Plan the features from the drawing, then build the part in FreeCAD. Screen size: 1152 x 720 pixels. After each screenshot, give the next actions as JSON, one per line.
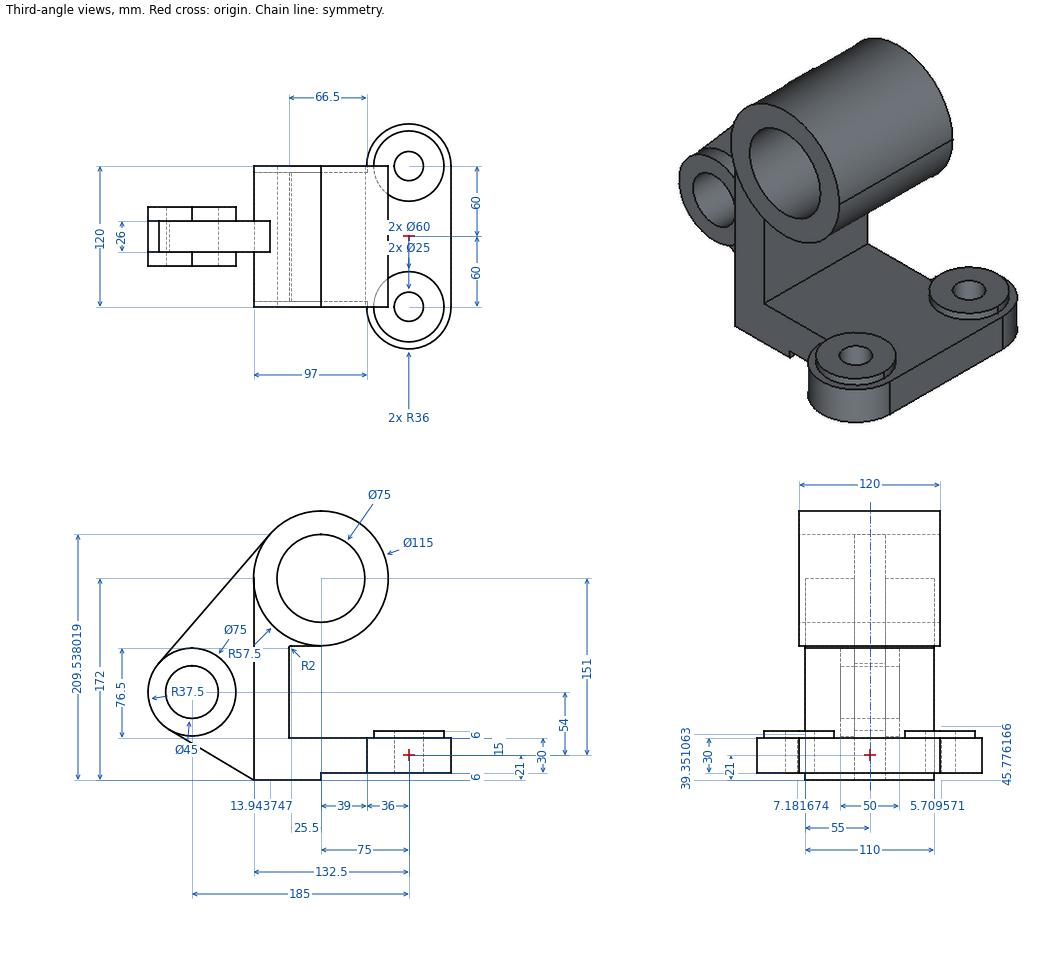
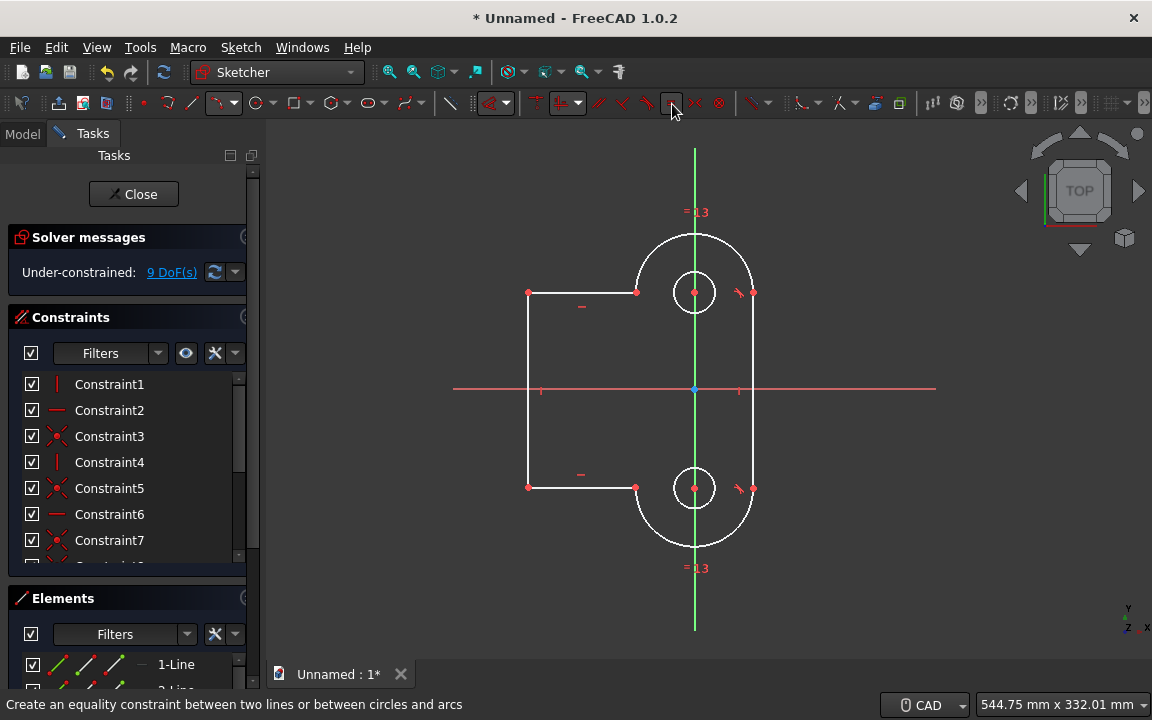
{"action": "left_click", "coordinate": [709, 474]}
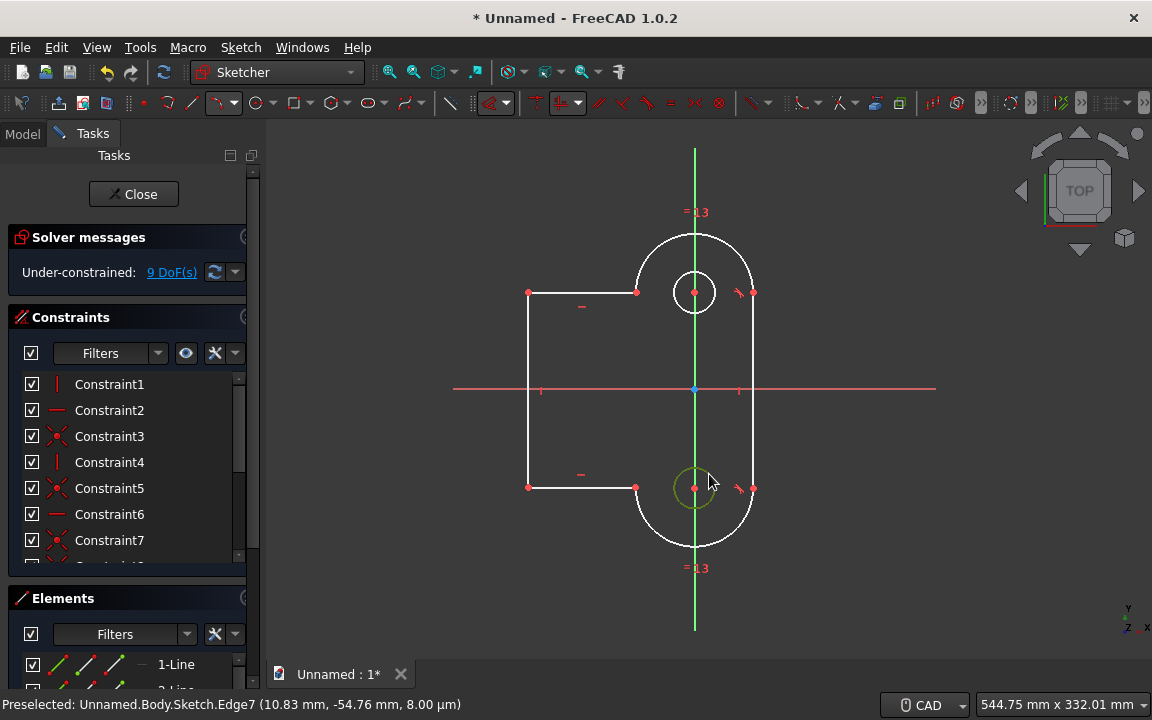
{"action": "left_click", "coordinate": [709, 278]}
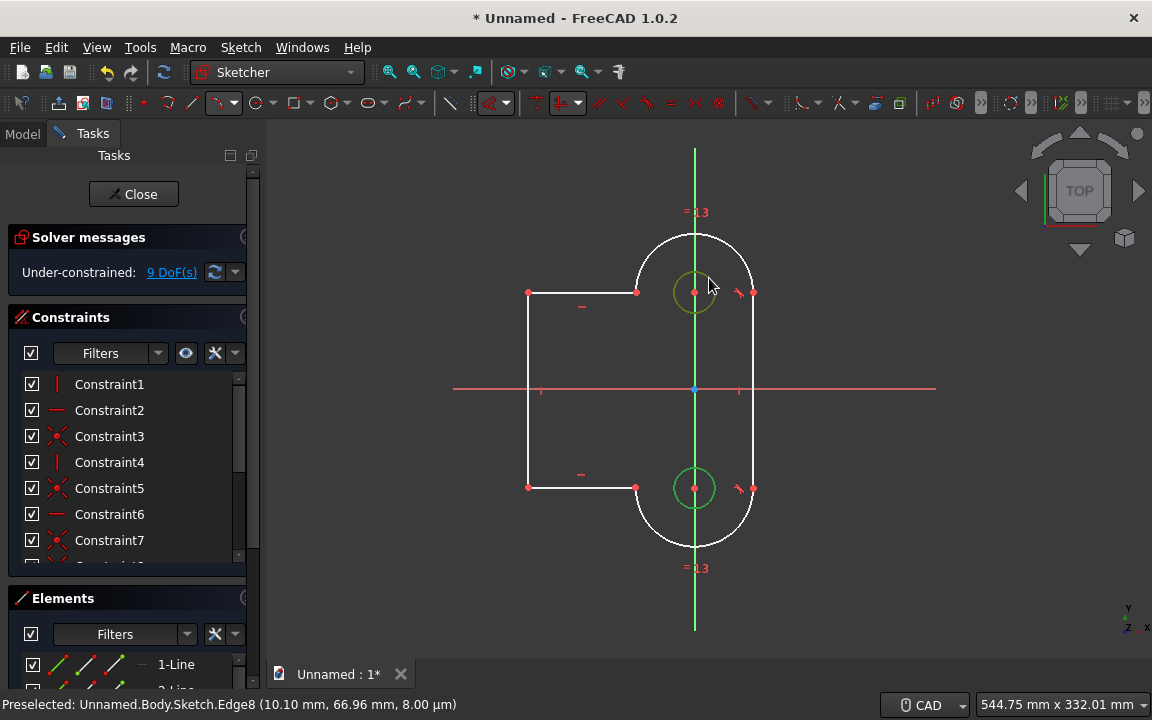
{"action": "left_click", "coordinate": [672, 104]}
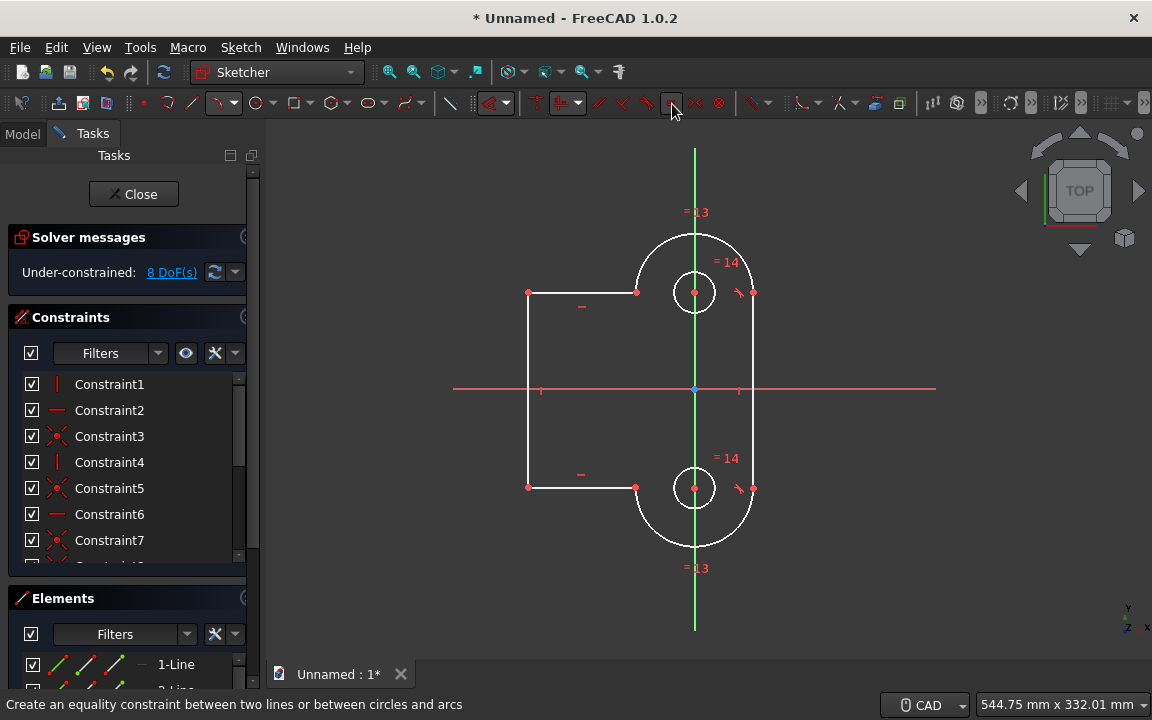
{"action": "left_click", "coordinate": [694, 293]}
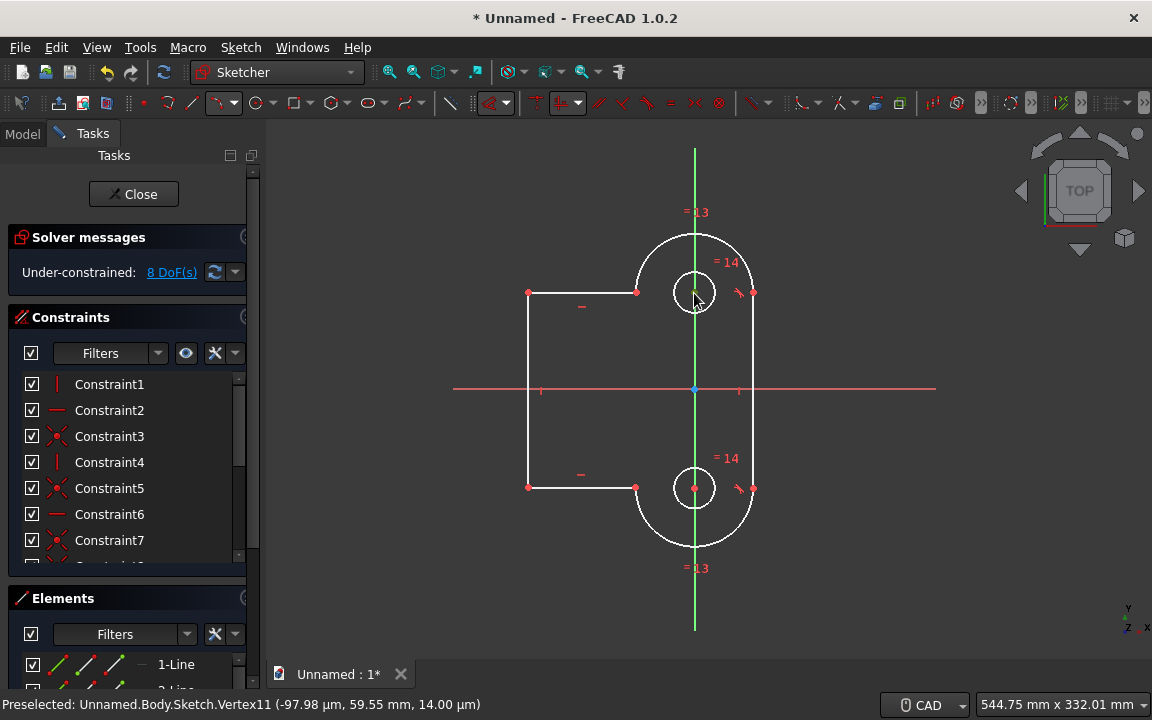
{"action": "left_click", "coordinate": [695, 596]}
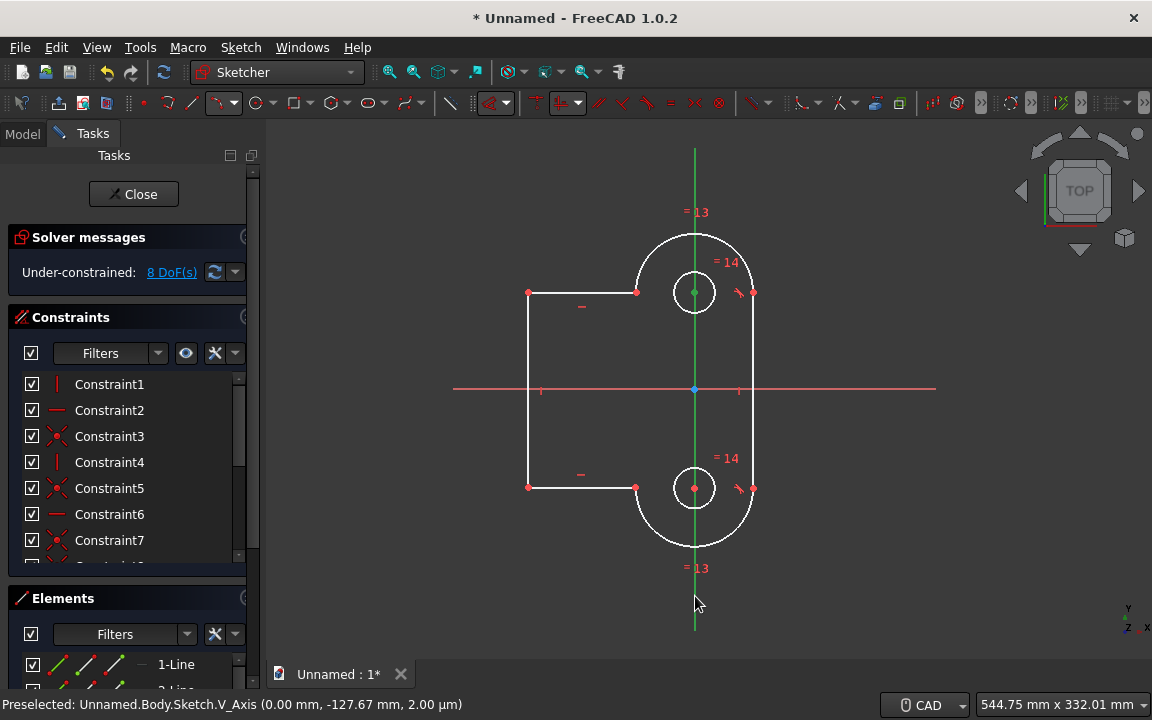
{"action": "key", "text": "c"}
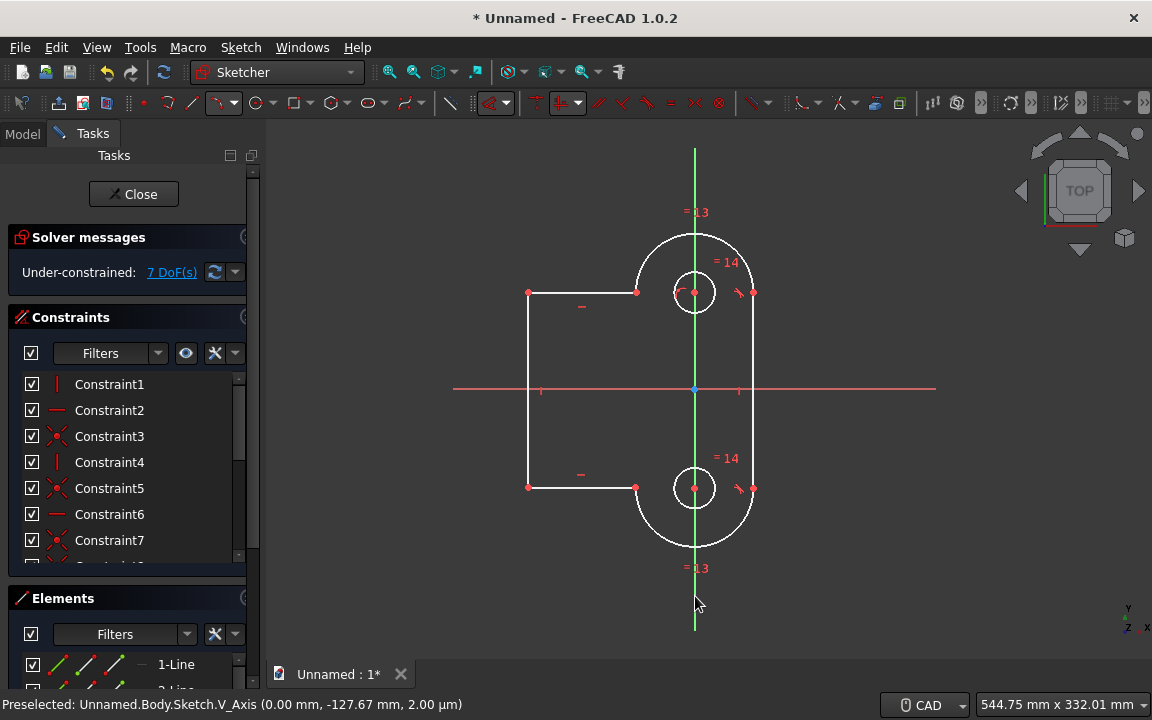
{"action": "left_click", "coordinate": [729, 245]}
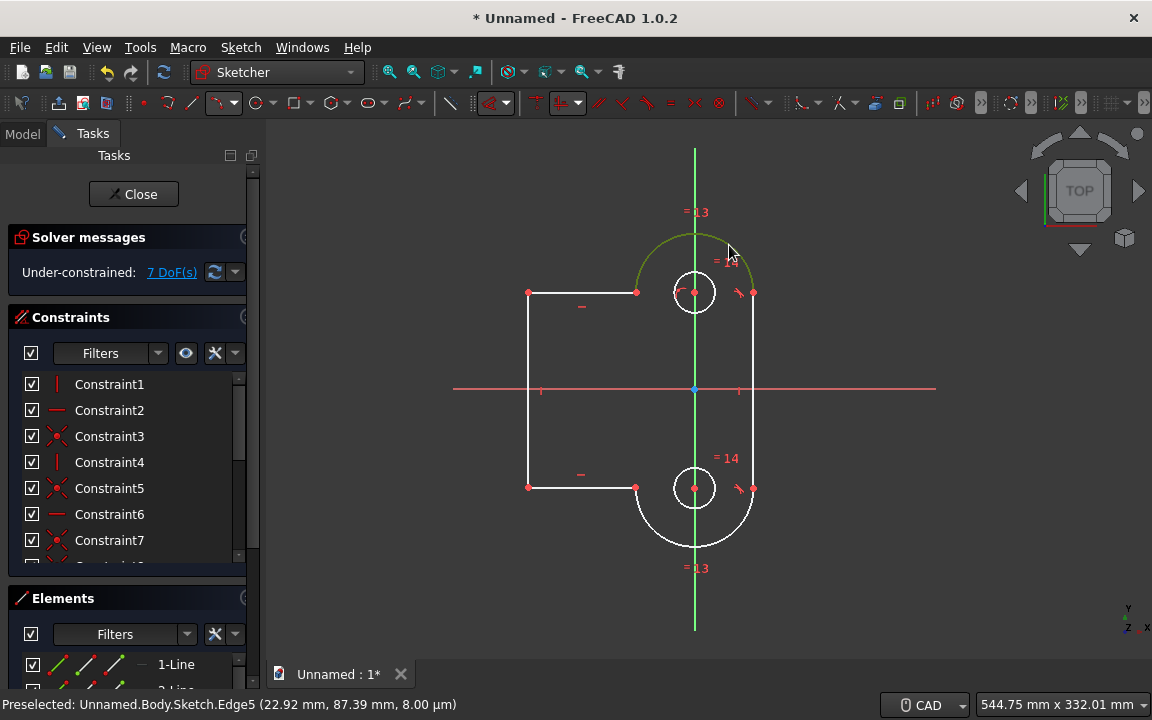
{"action": "key", "text": "k r"}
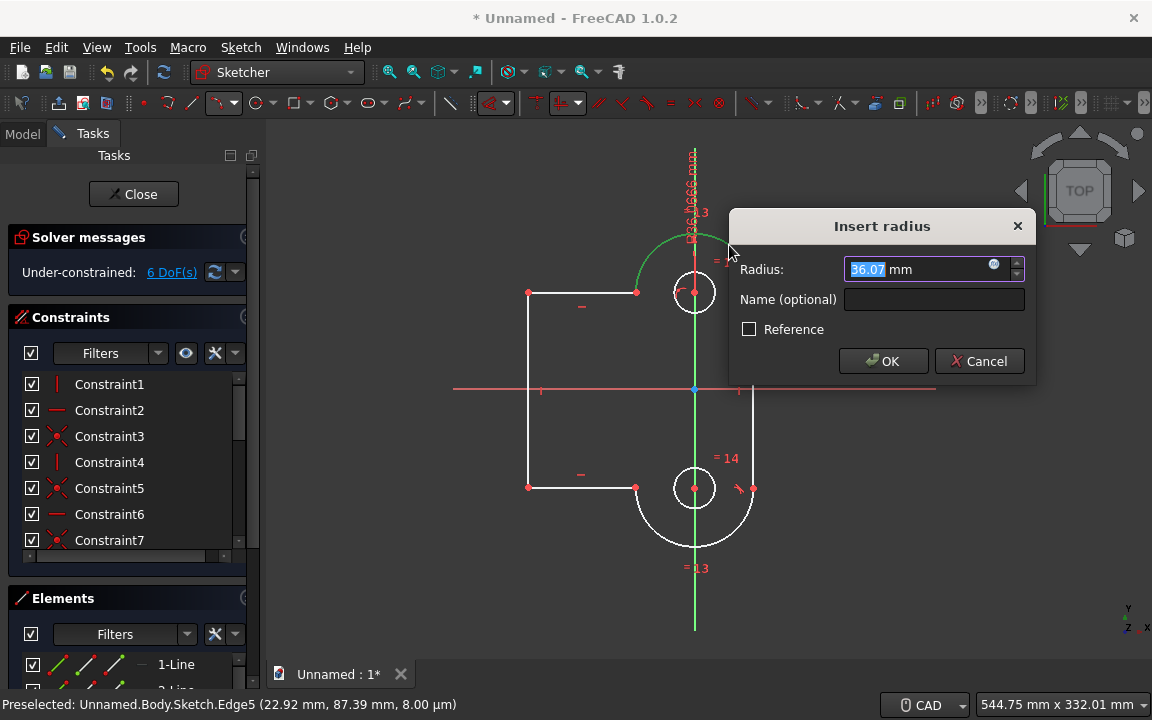
{"action": "type", "text": "36"}
{"action": "key", "text": "Return"}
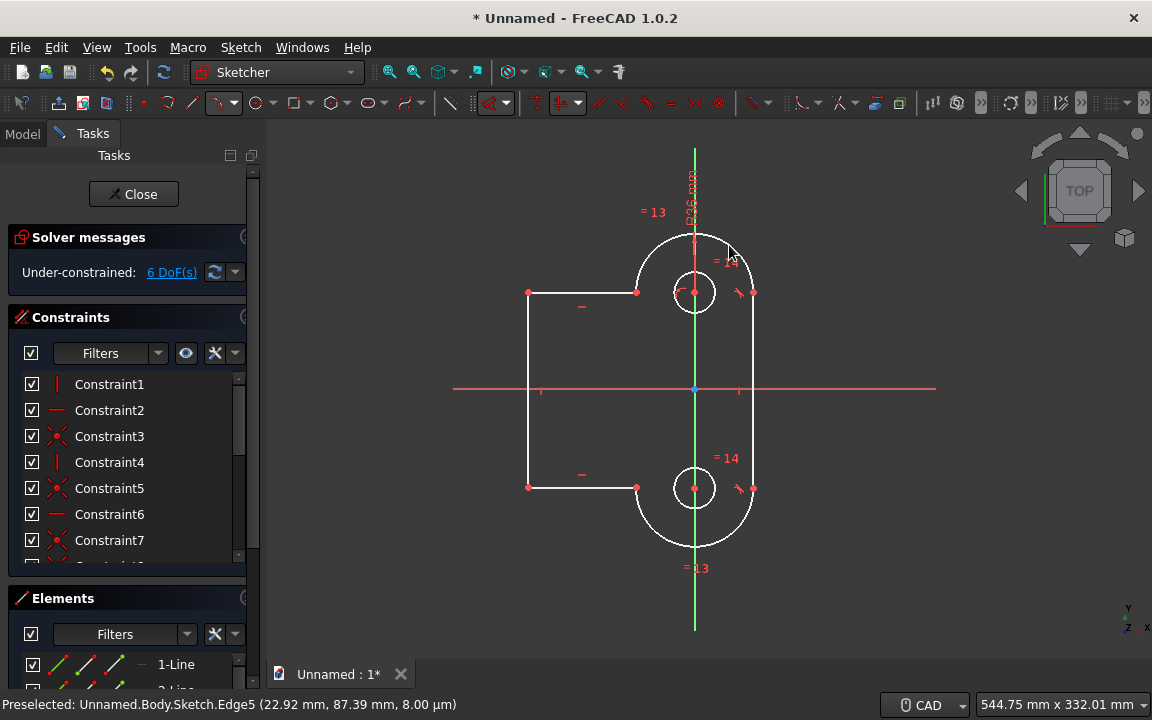
{"action": "left_click", "coordinate": [709, 474]}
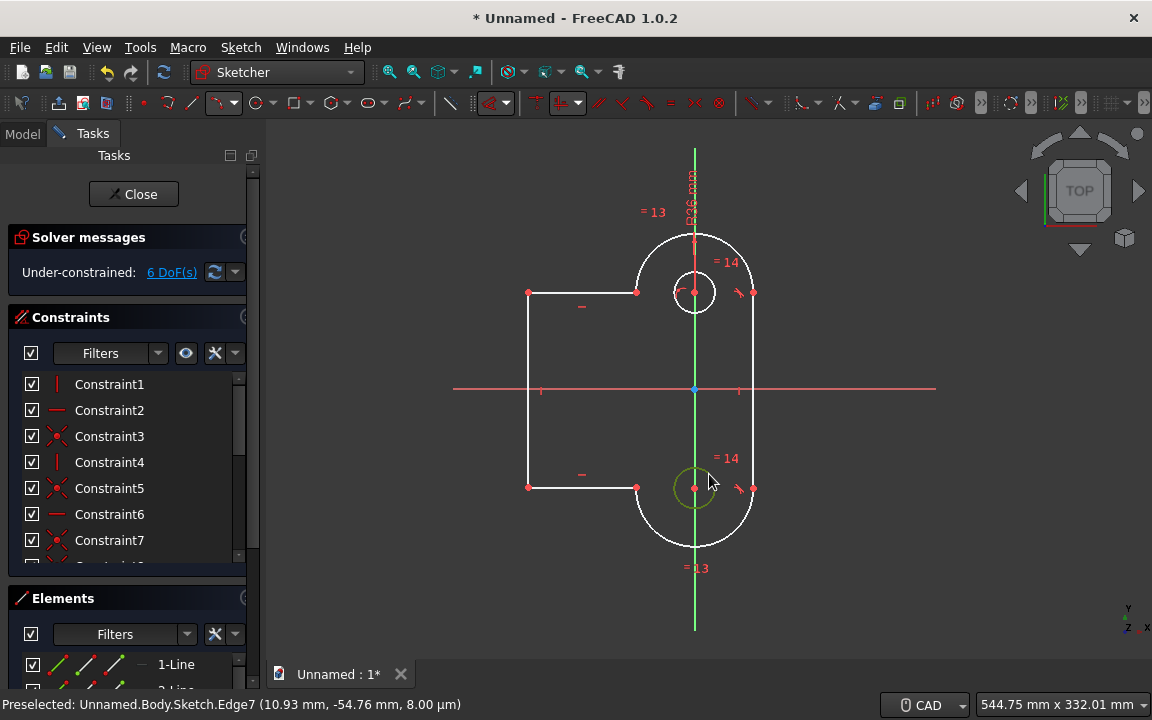
{"action": "left_click", "coordinate": [508, 104]}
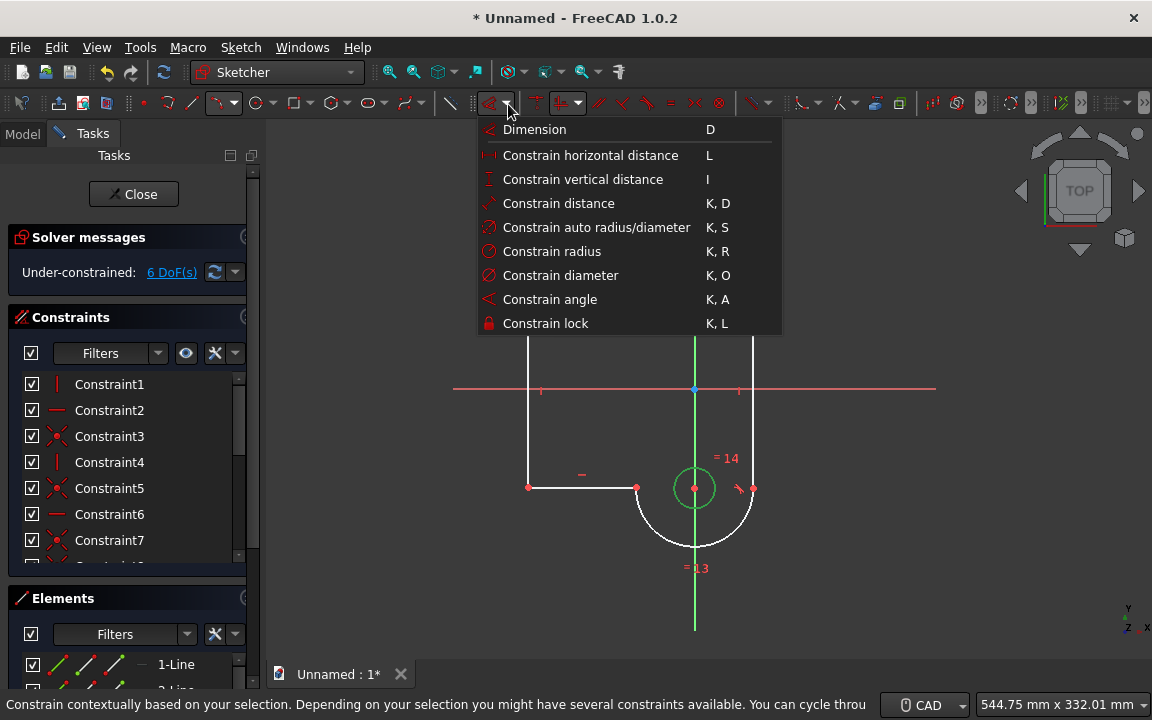
{"action": "left_click", "coordinate": [630, 275]}